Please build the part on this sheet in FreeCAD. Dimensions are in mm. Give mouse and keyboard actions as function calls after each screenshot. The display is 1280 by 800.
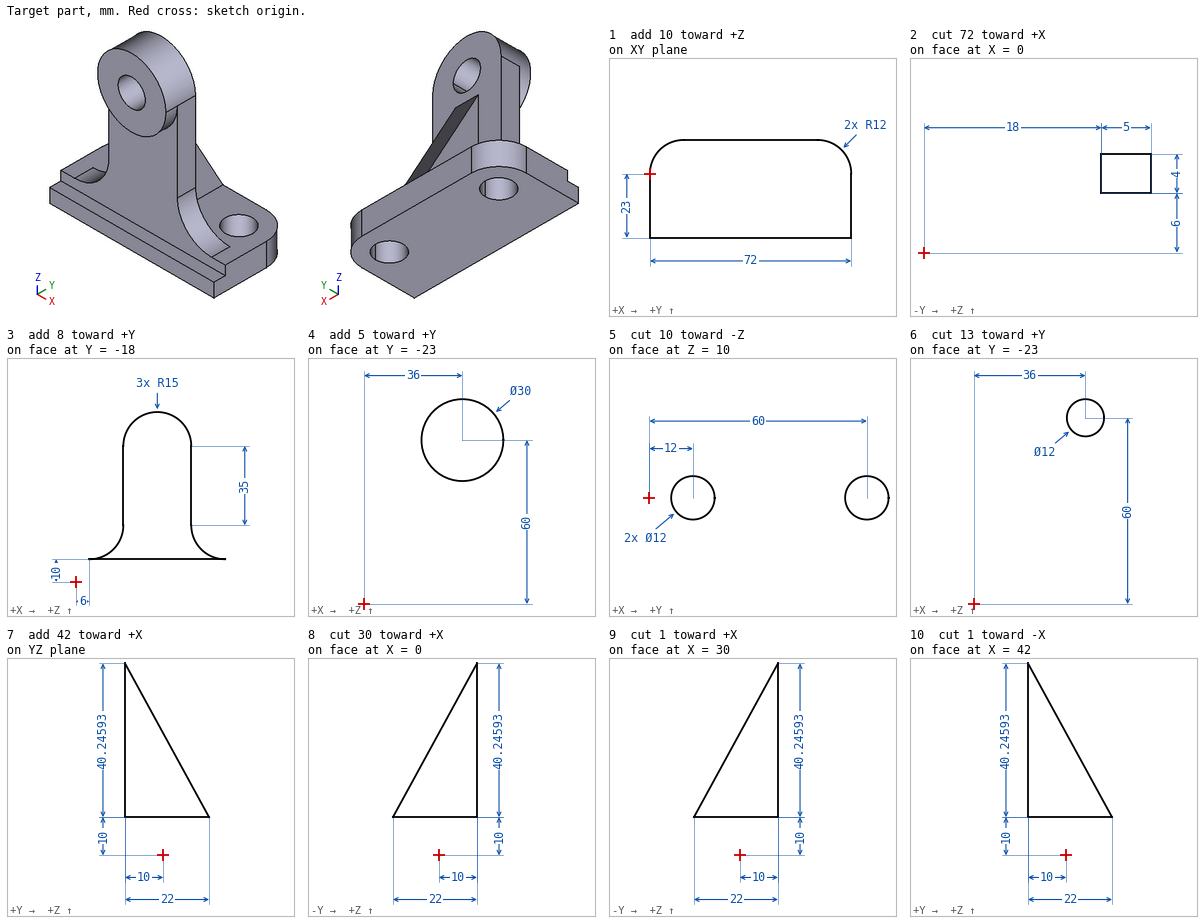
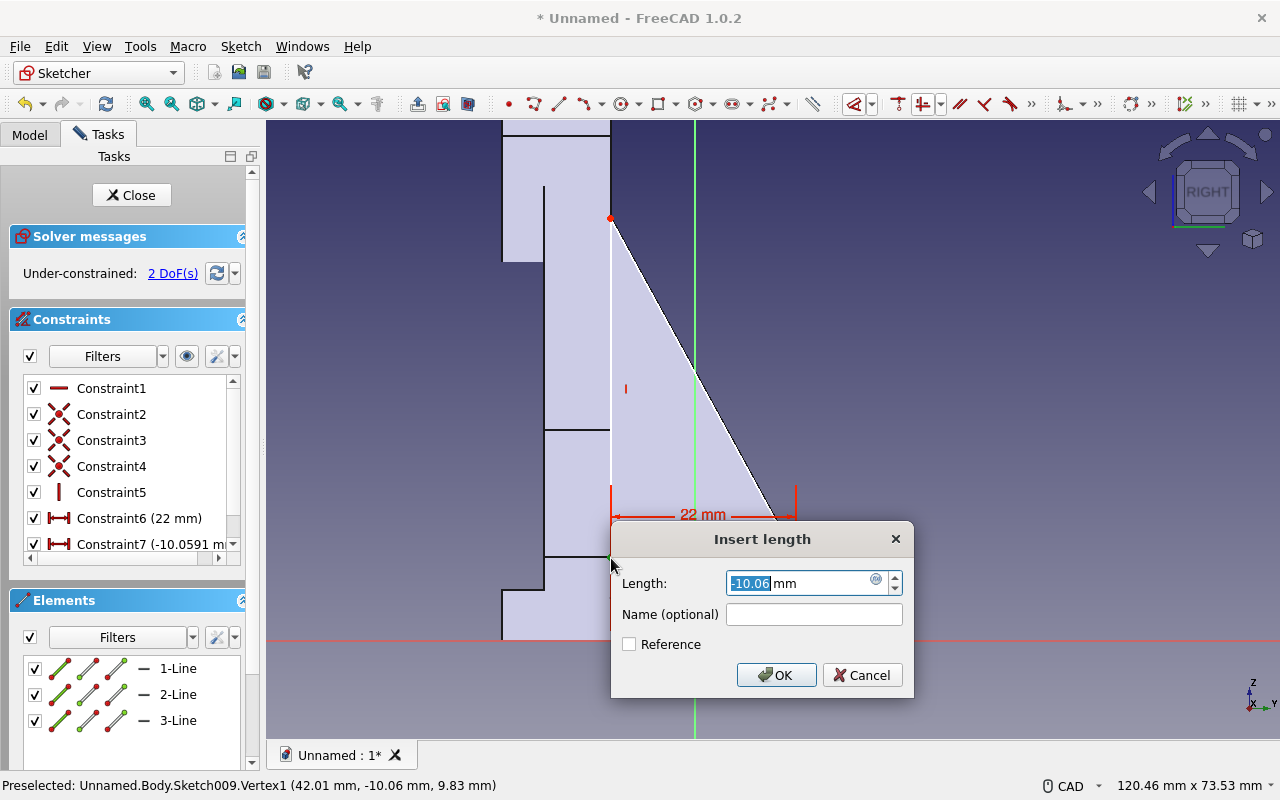
text(-10)
key(Return)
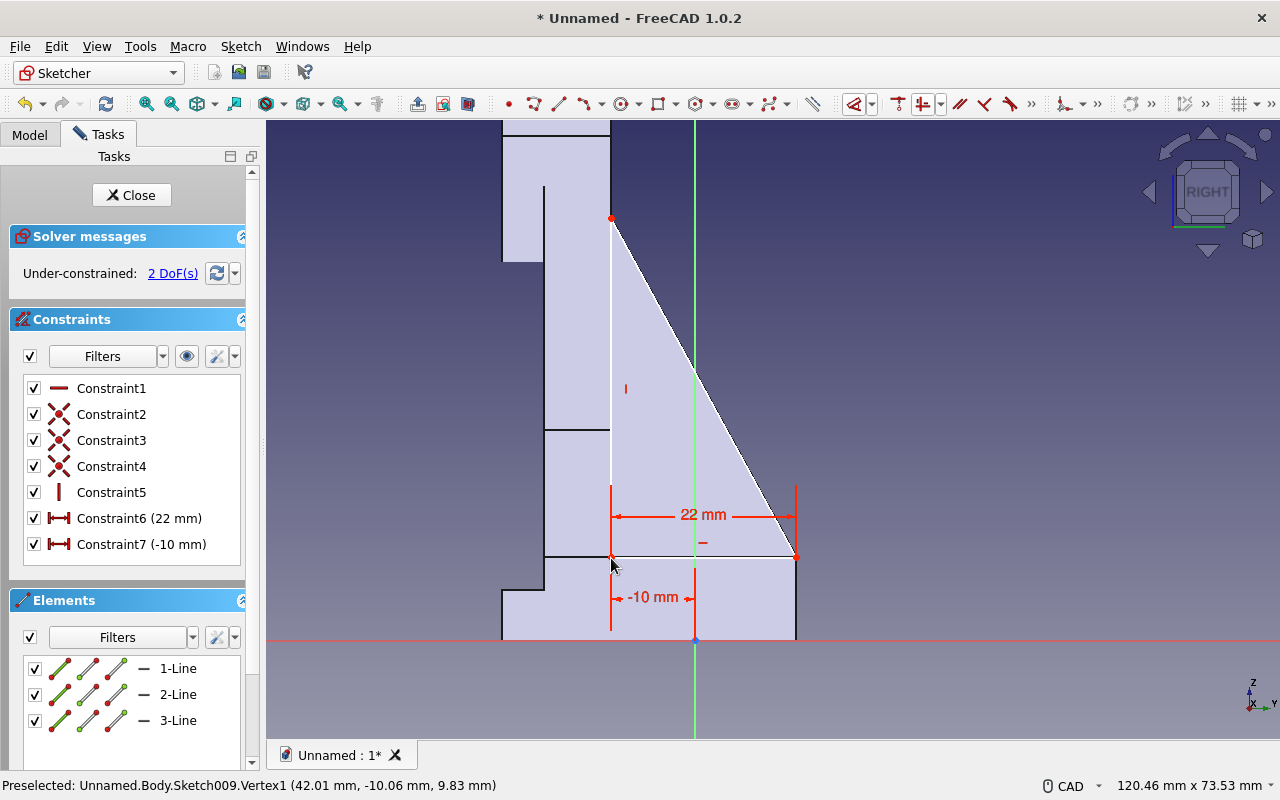
click(611, 558)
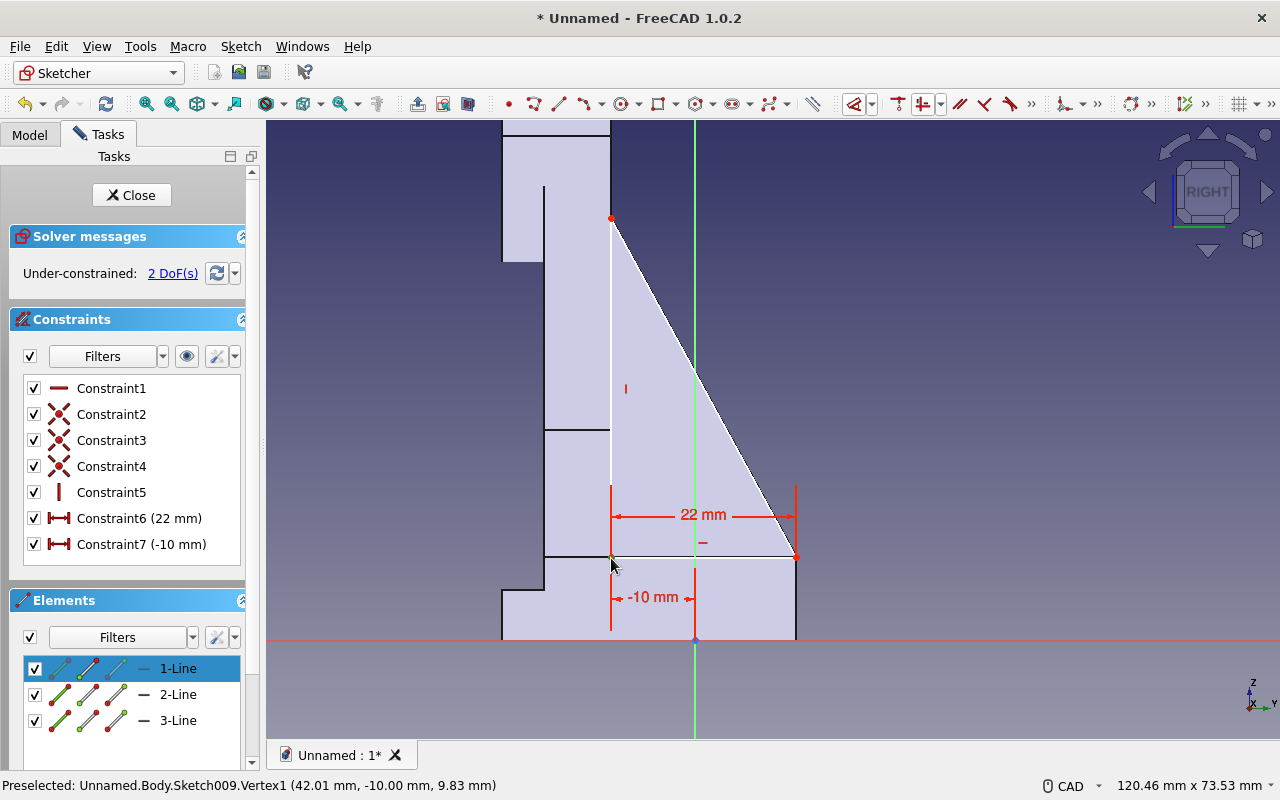
click(872, 104)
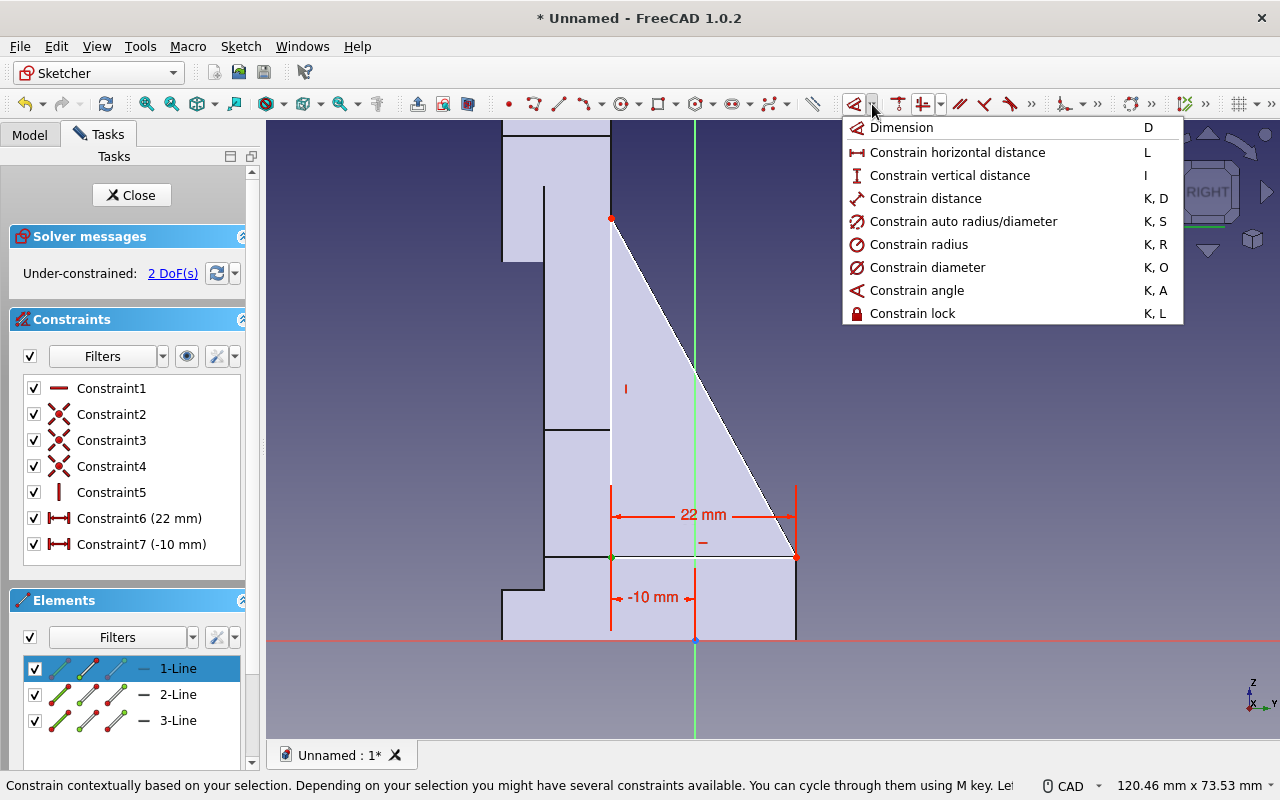
click(1013, 176)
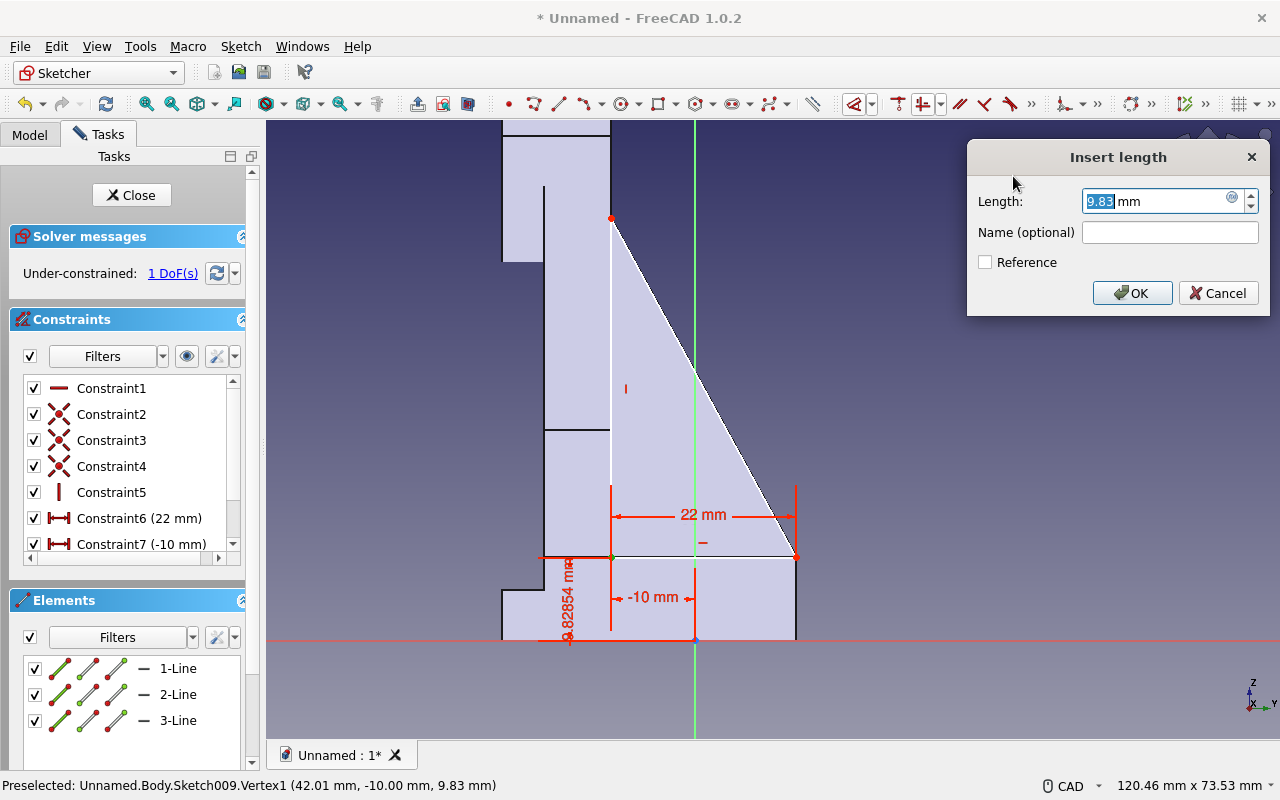
text(10)
key(Return)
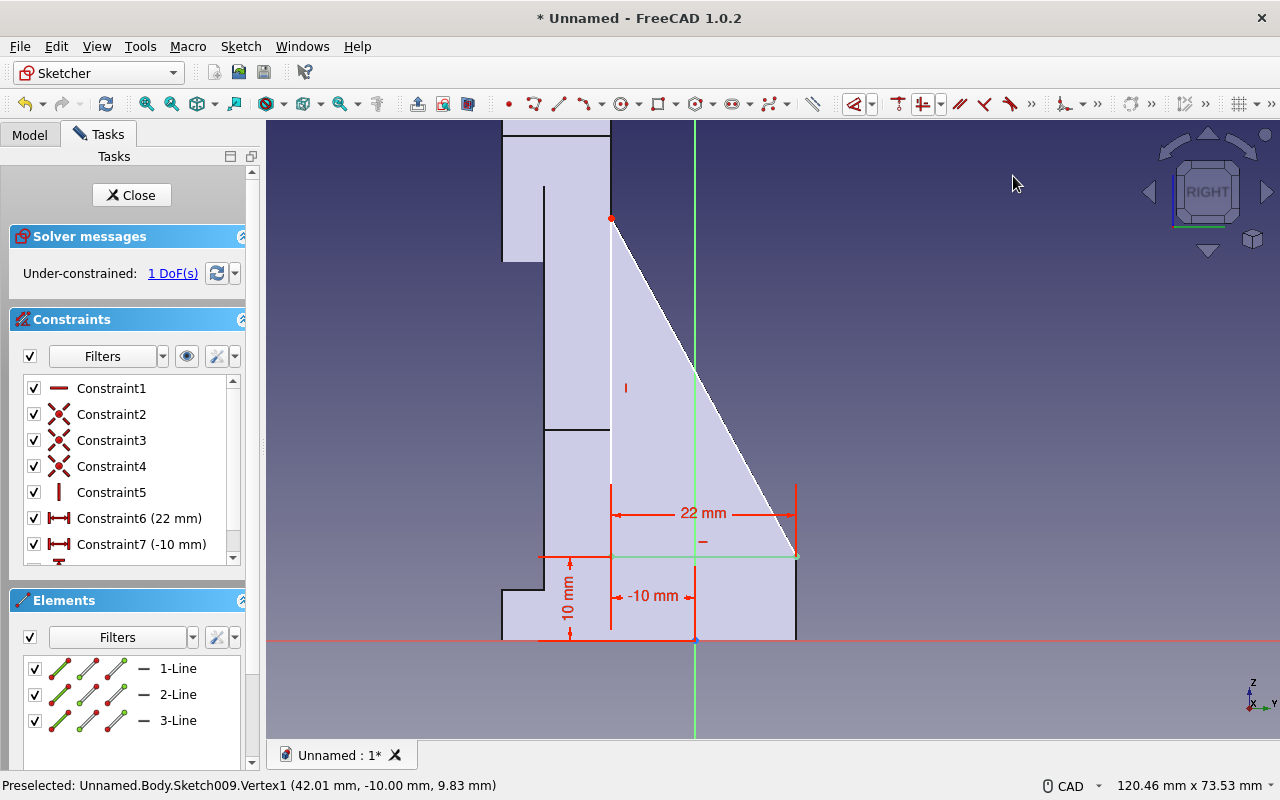
click(611, 320)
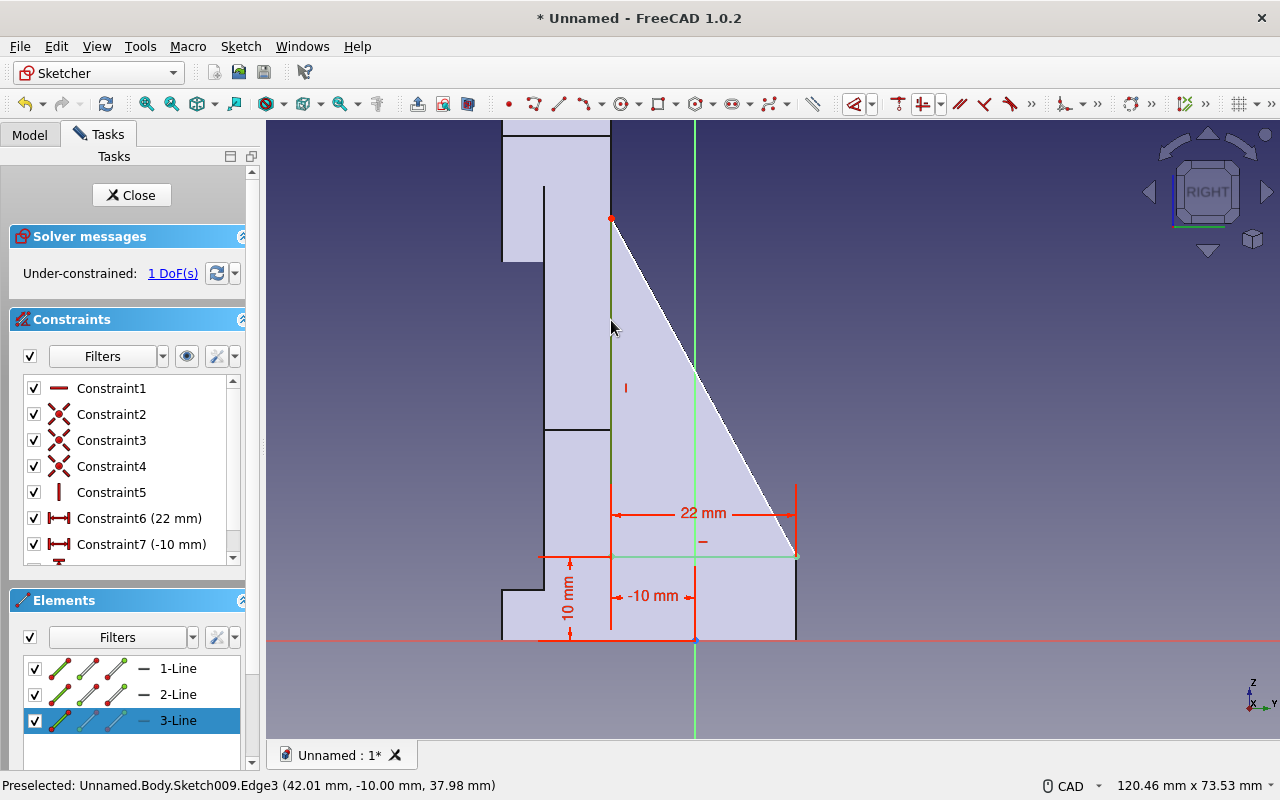
click(872, 104)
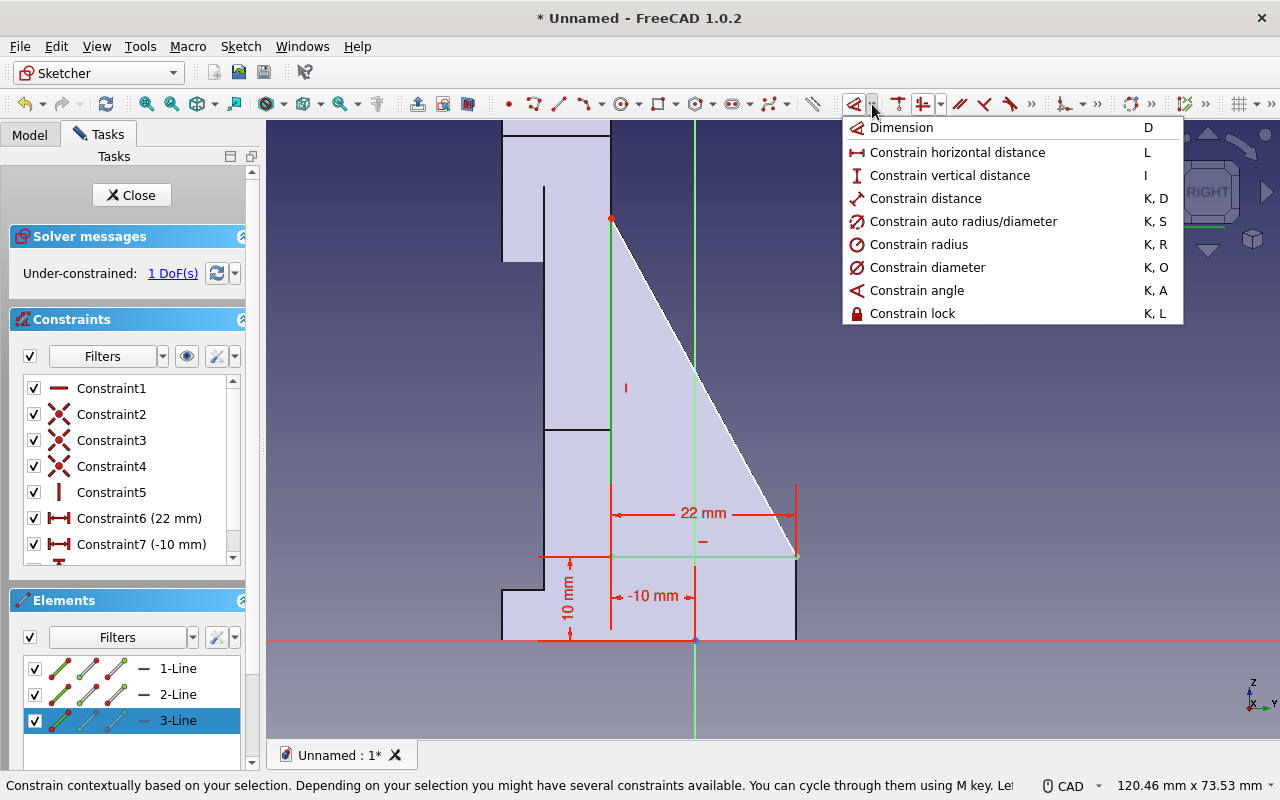
click(1013, 176)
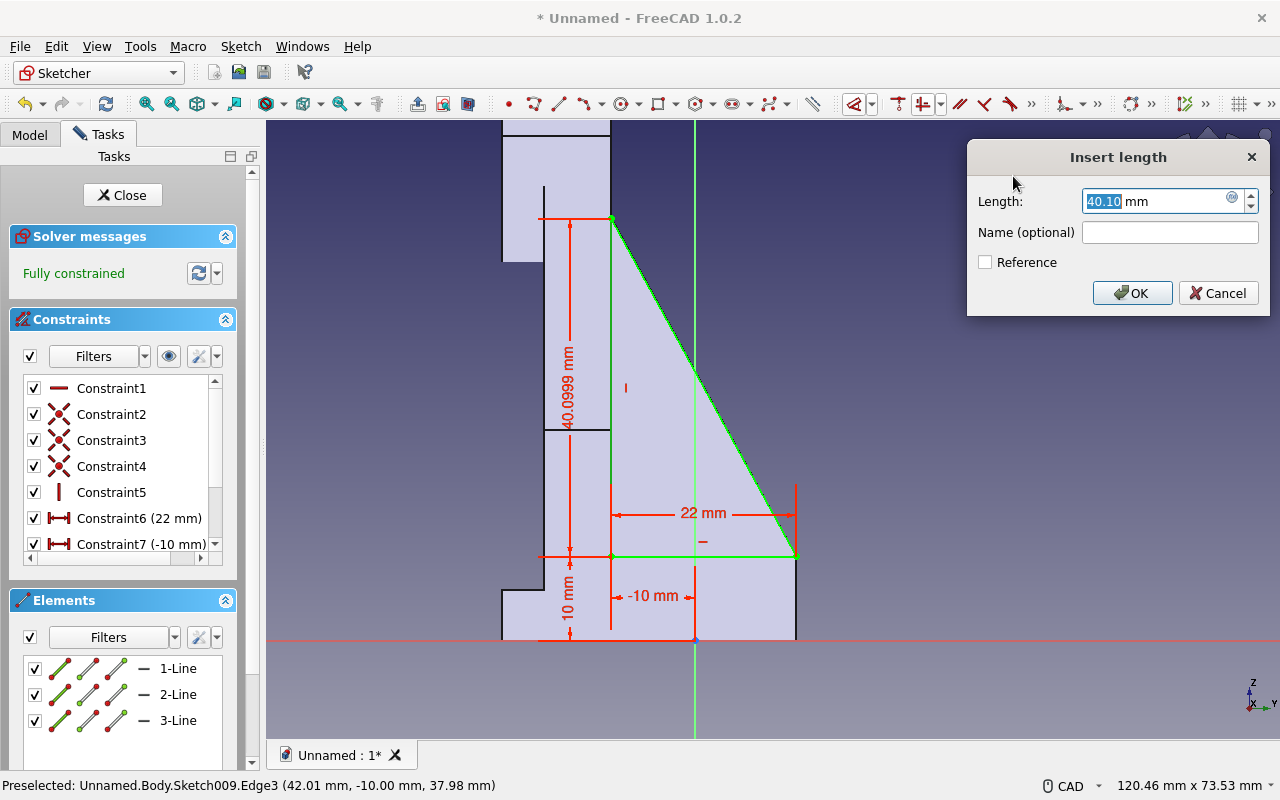
text(40.24593)
key(Return)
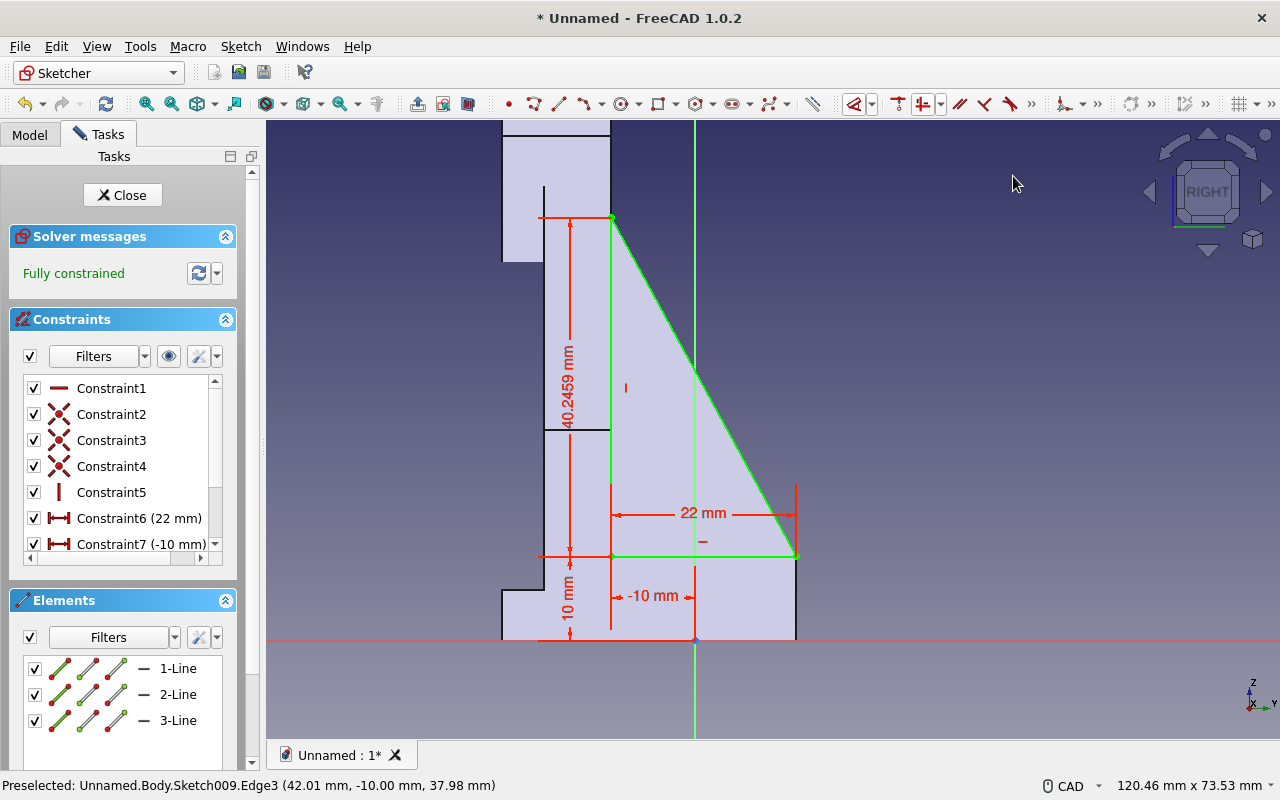
click(123, 195)